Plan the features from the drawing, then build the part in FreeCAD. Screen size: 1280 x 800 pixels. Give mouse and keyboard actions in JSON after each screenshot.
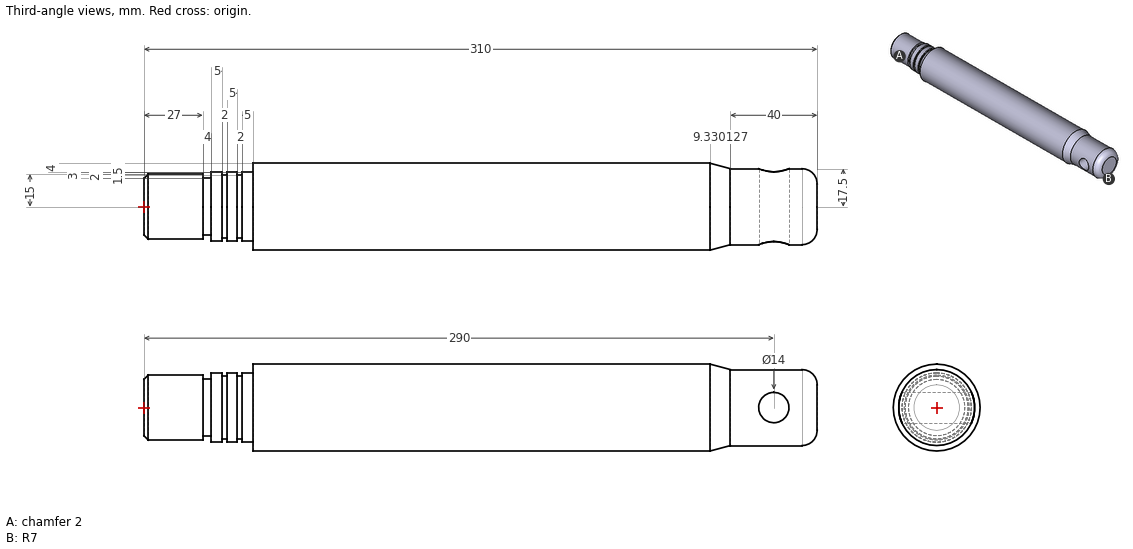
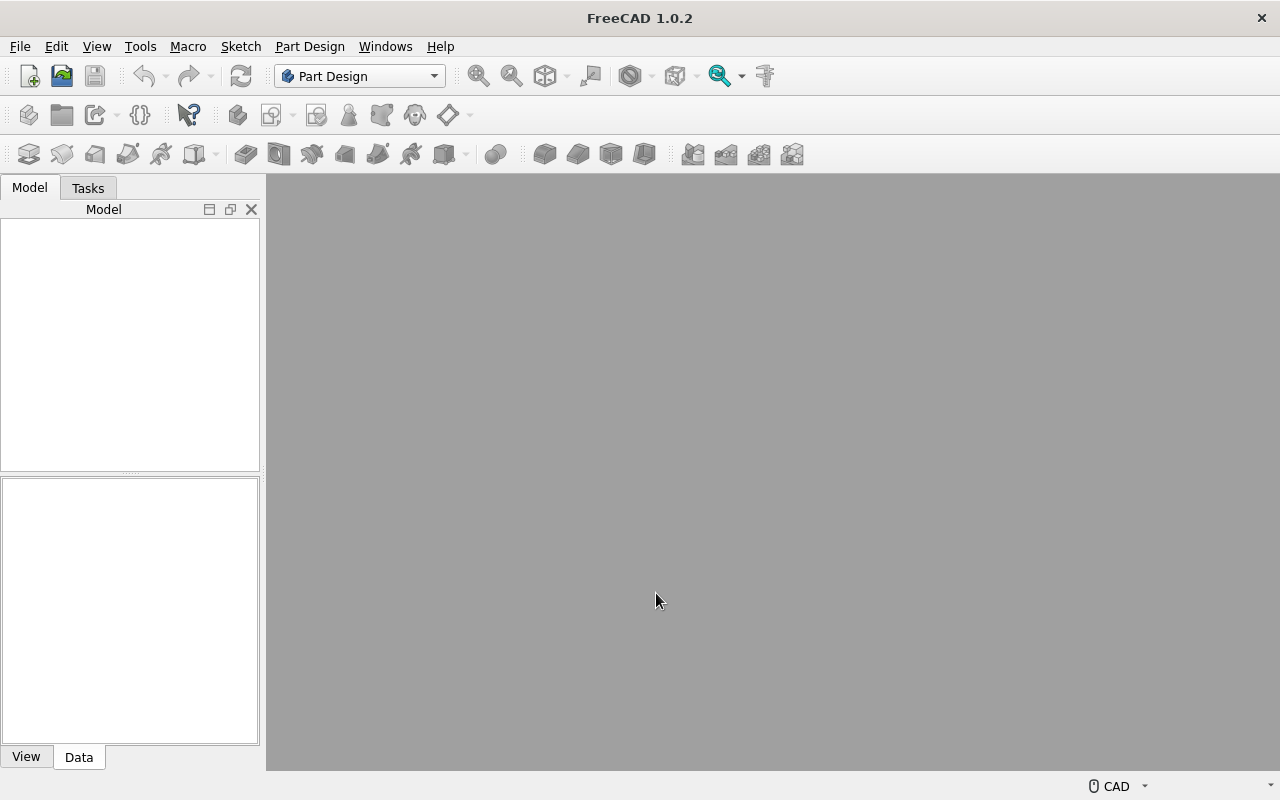
{"action": "key", "text": "ctrl+n"}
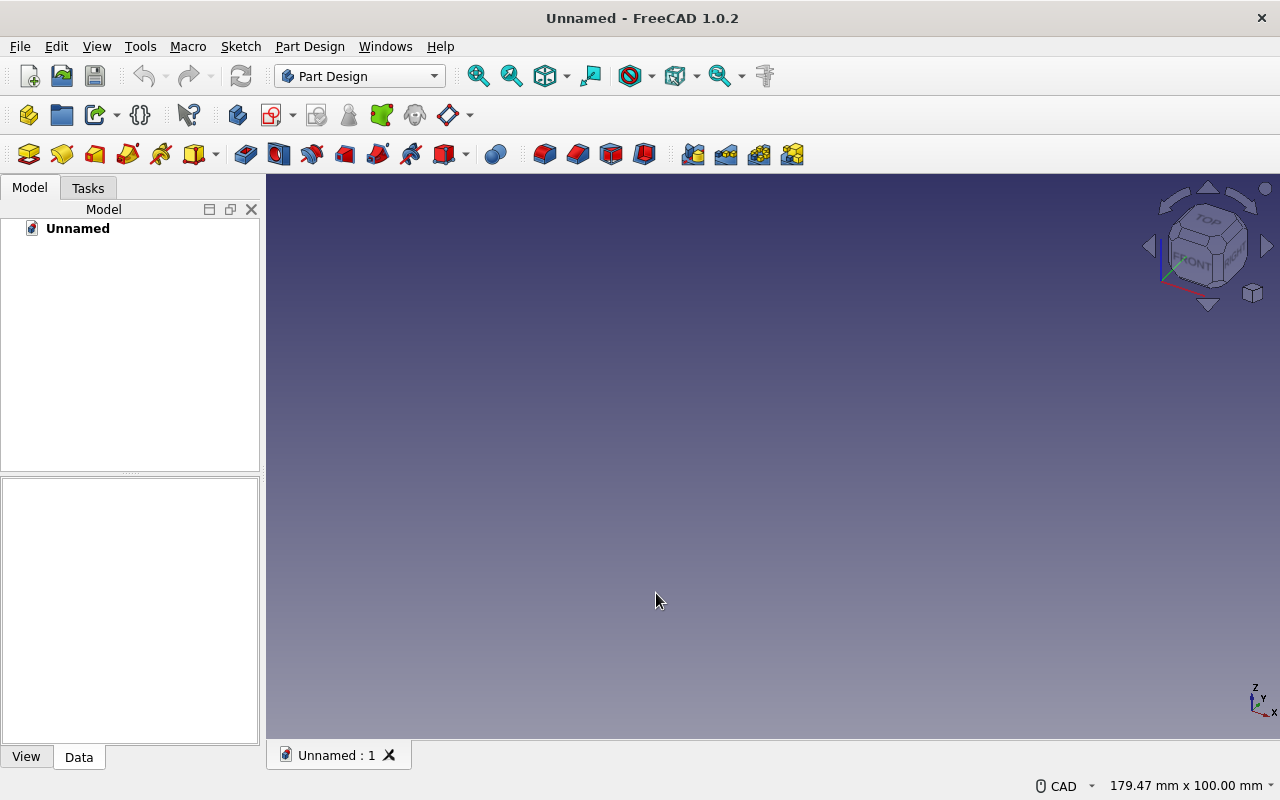
{"action": "left_click", "coordinate": [270, 116]}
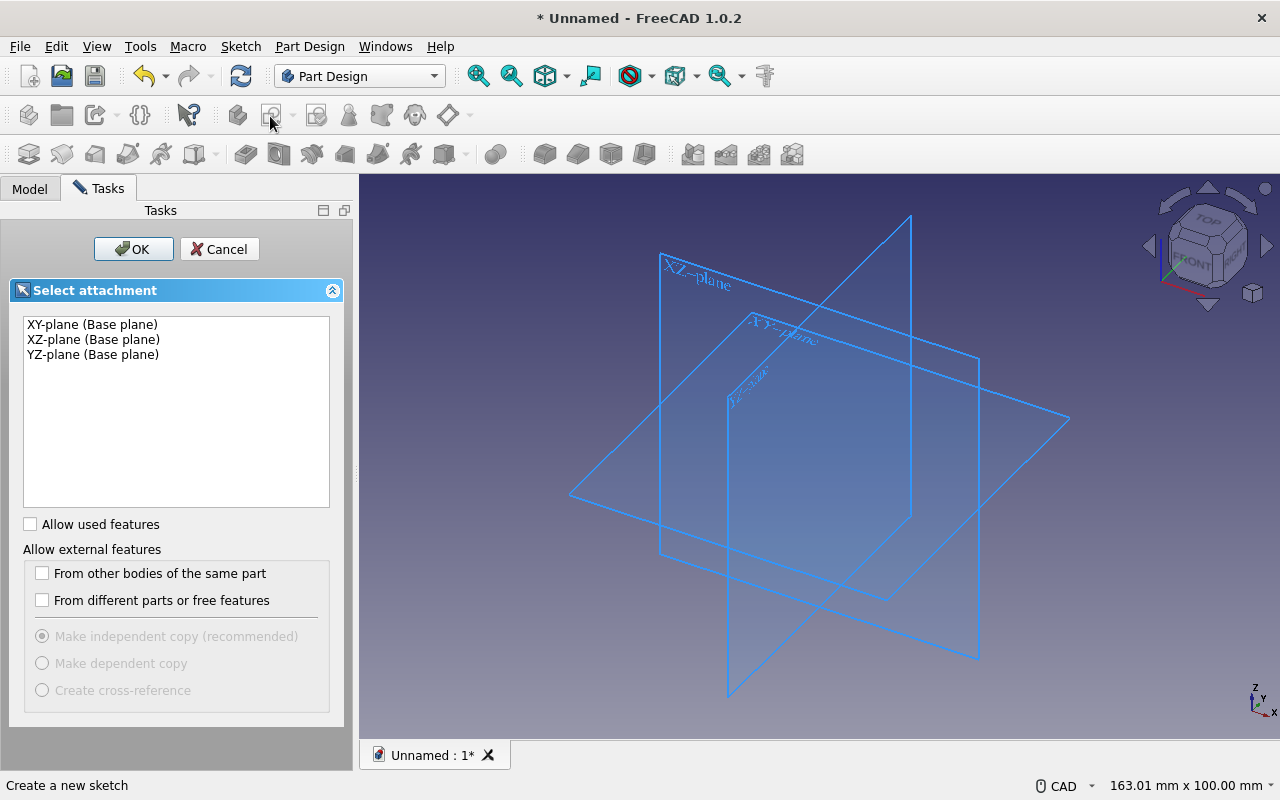
{"action": "left_click", "coordinate": [84, 324]}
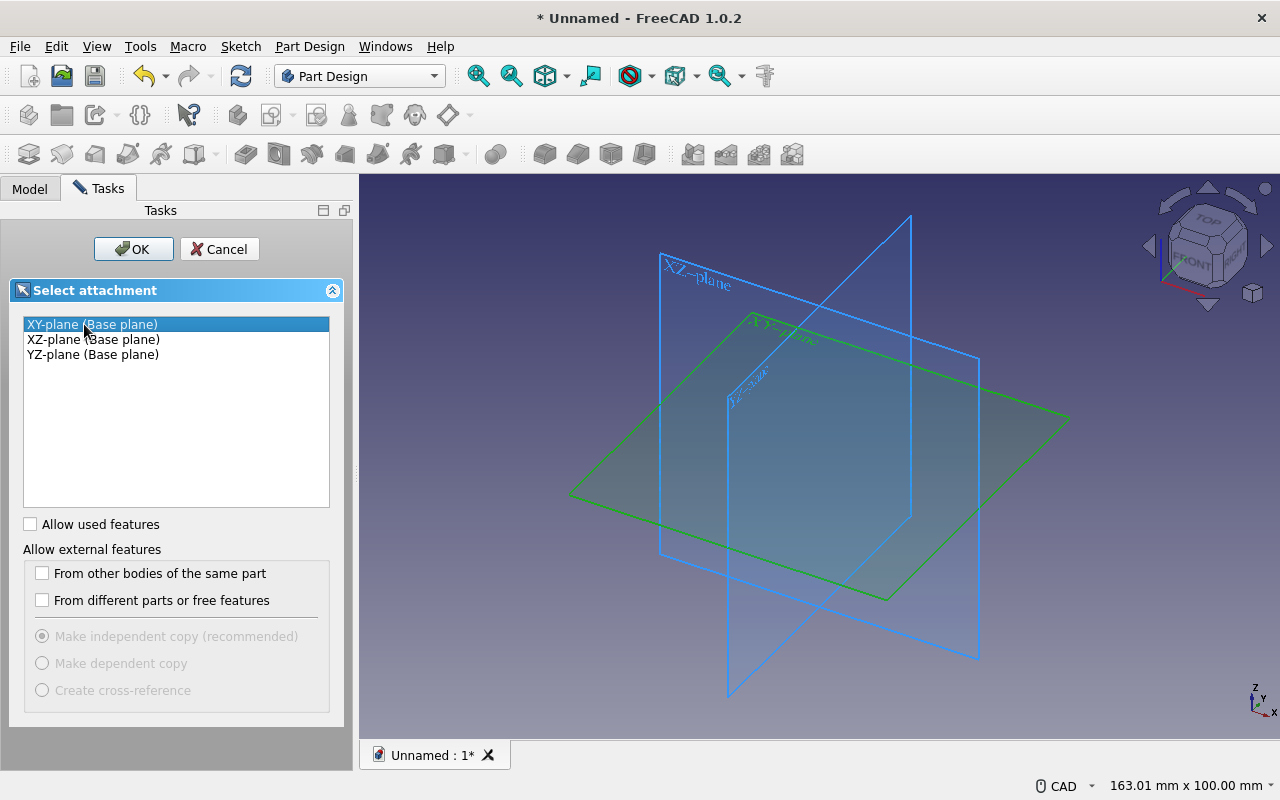
{"action": "left_click", "coordinate": [134, 249]}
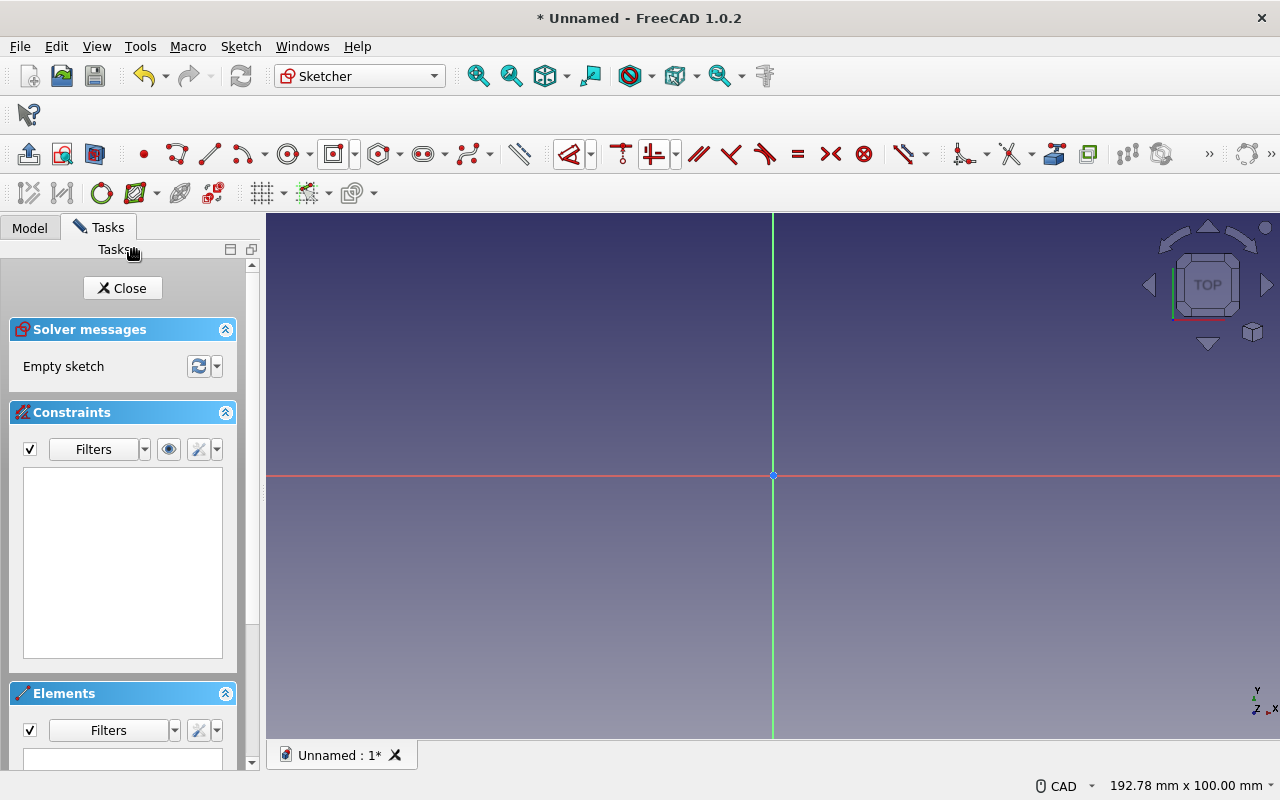
{"action": "scroll", "coordinate": [294, 507], "scroll_direction": "down", "scroll_amount": 5}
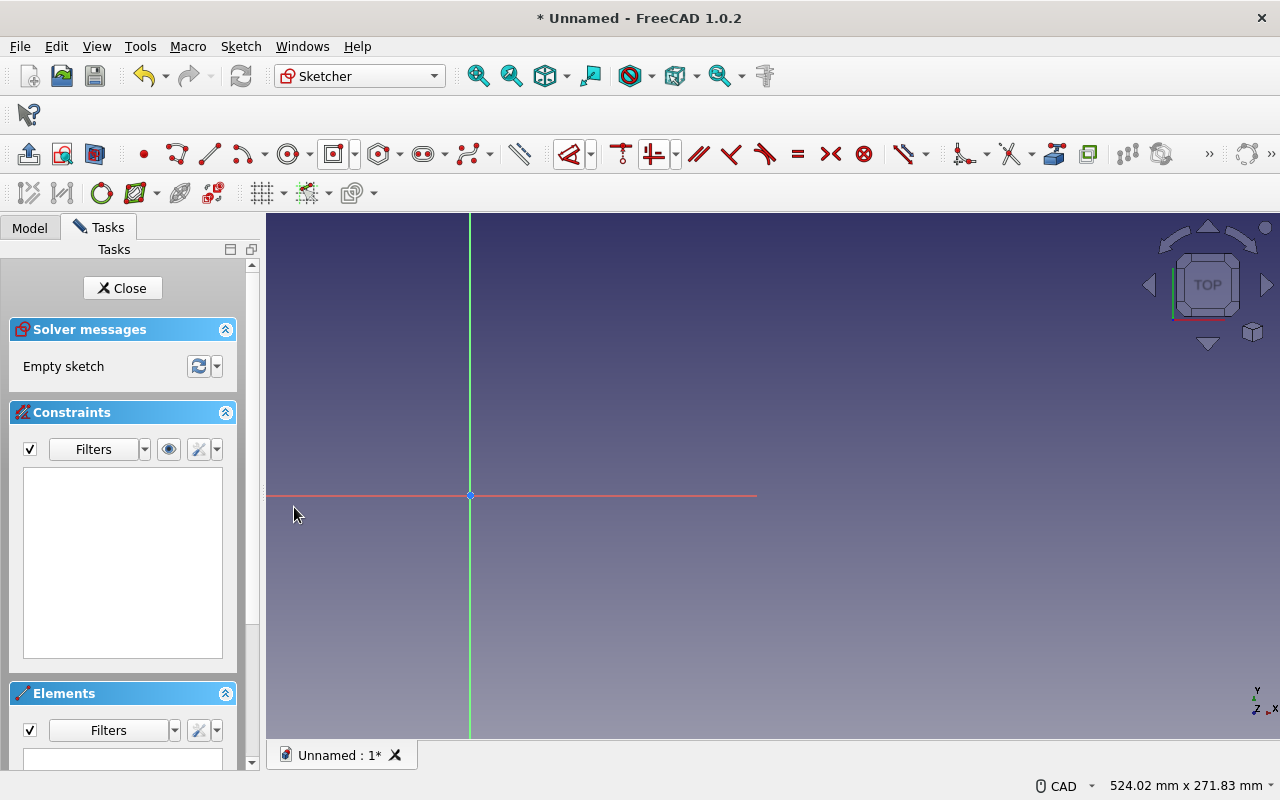
{"action": "left_click", "coordinate": [177, 154]}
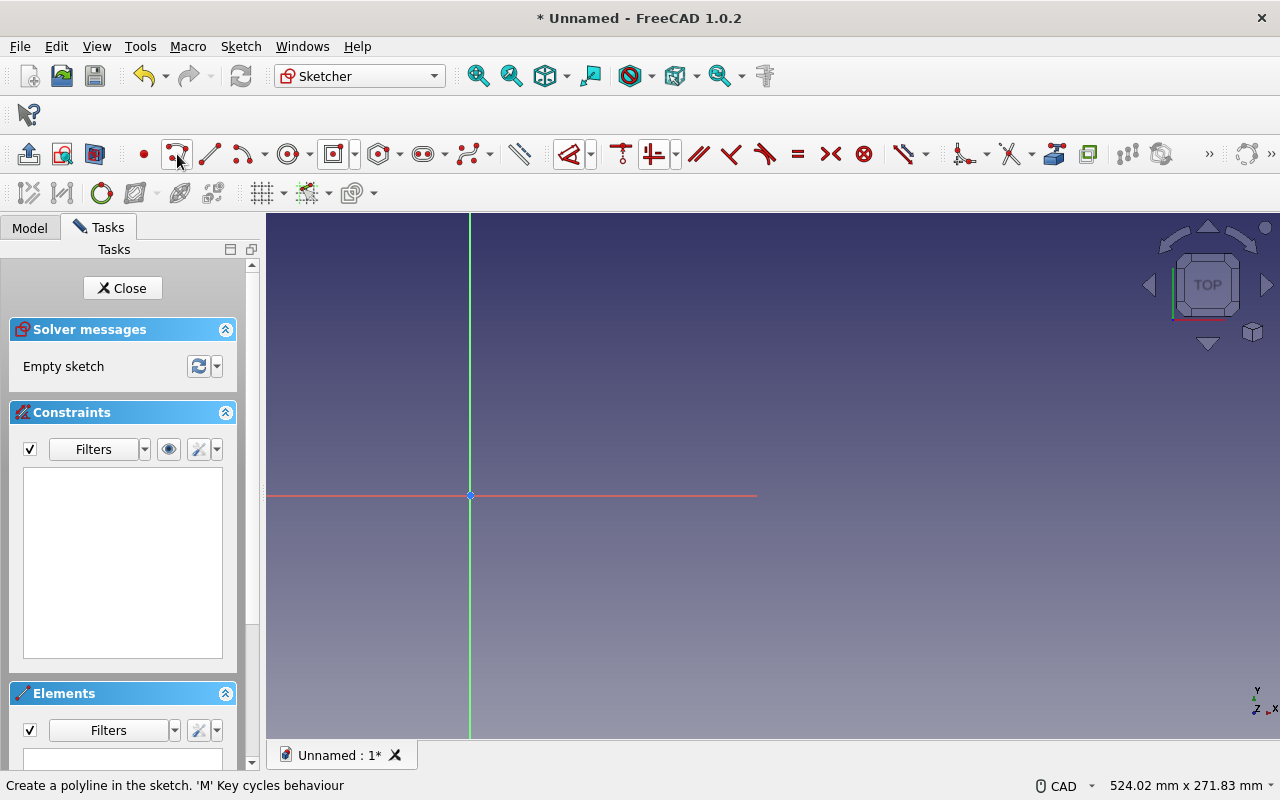
{"action": "left_click", "coordinate": [470, 496]}
{"action": "left_click", "coordinate": [1070, 487]}
{"action": "left_click", "coordinate": [1070, 462]}
{"action": "left_click", "coordinate": [993, 462]}
{"action": "left_click", "coordinate": [975, 457]}
{"action": "left_click", "coordinate": [567, 457]}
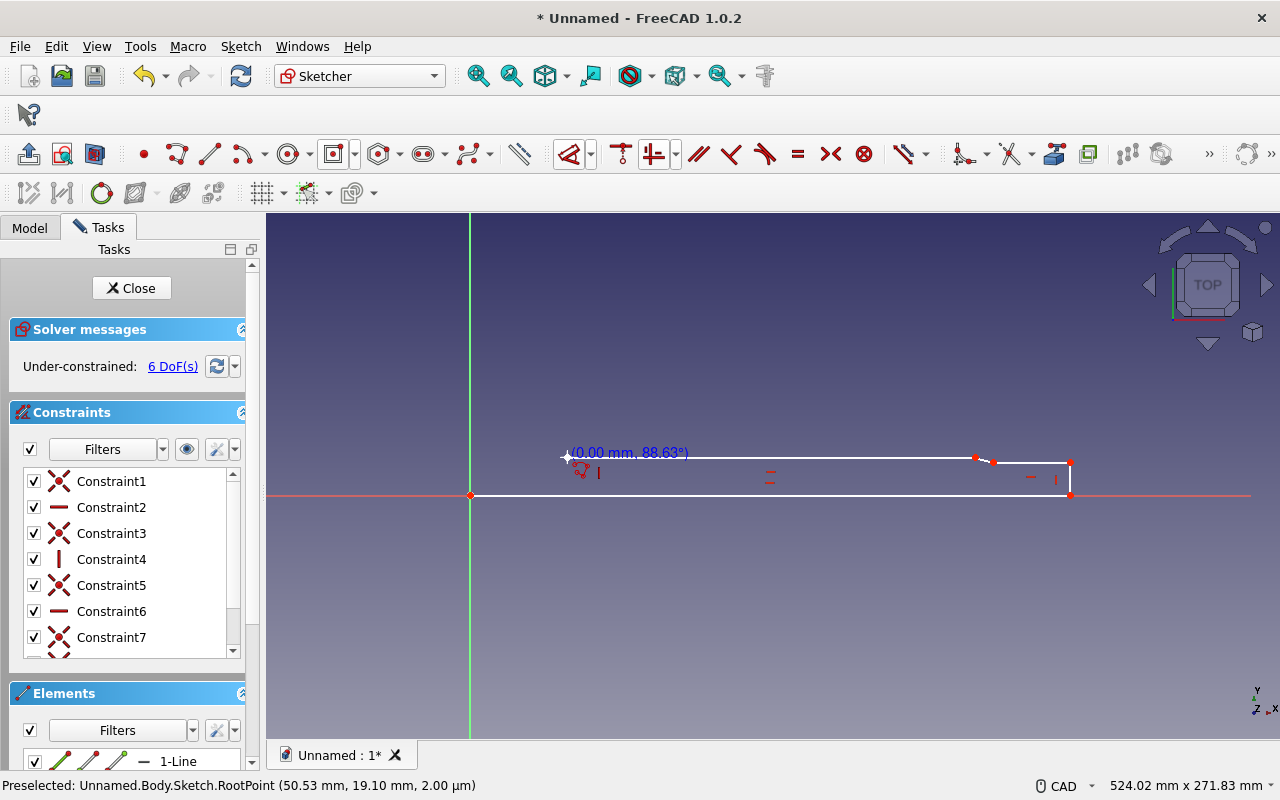
{"action": "scroll", "coordinate": [567, 465], "scroll_direction": "up", "scroll_amount": 4}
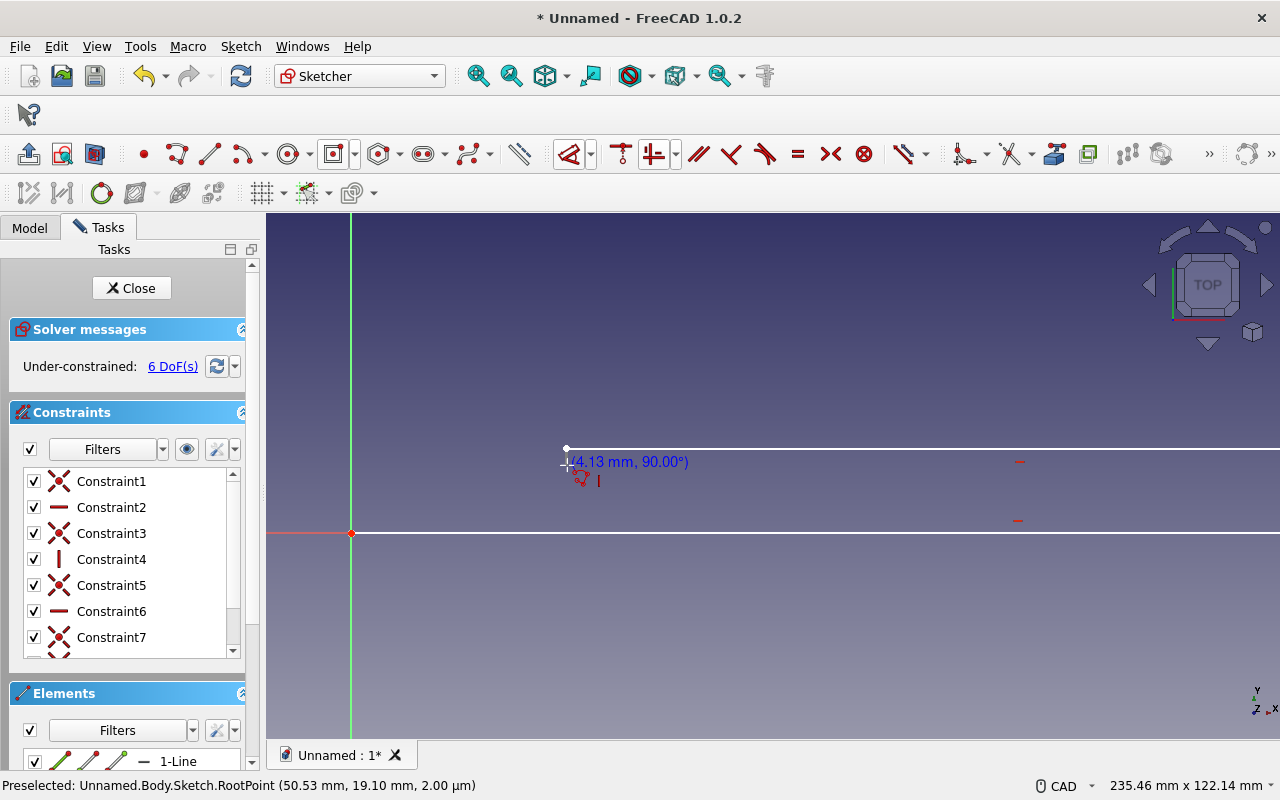
{"action": "left_click", "coordinate": [567, 464]}
{"action": "left_click", "coordinate": [545, 464]}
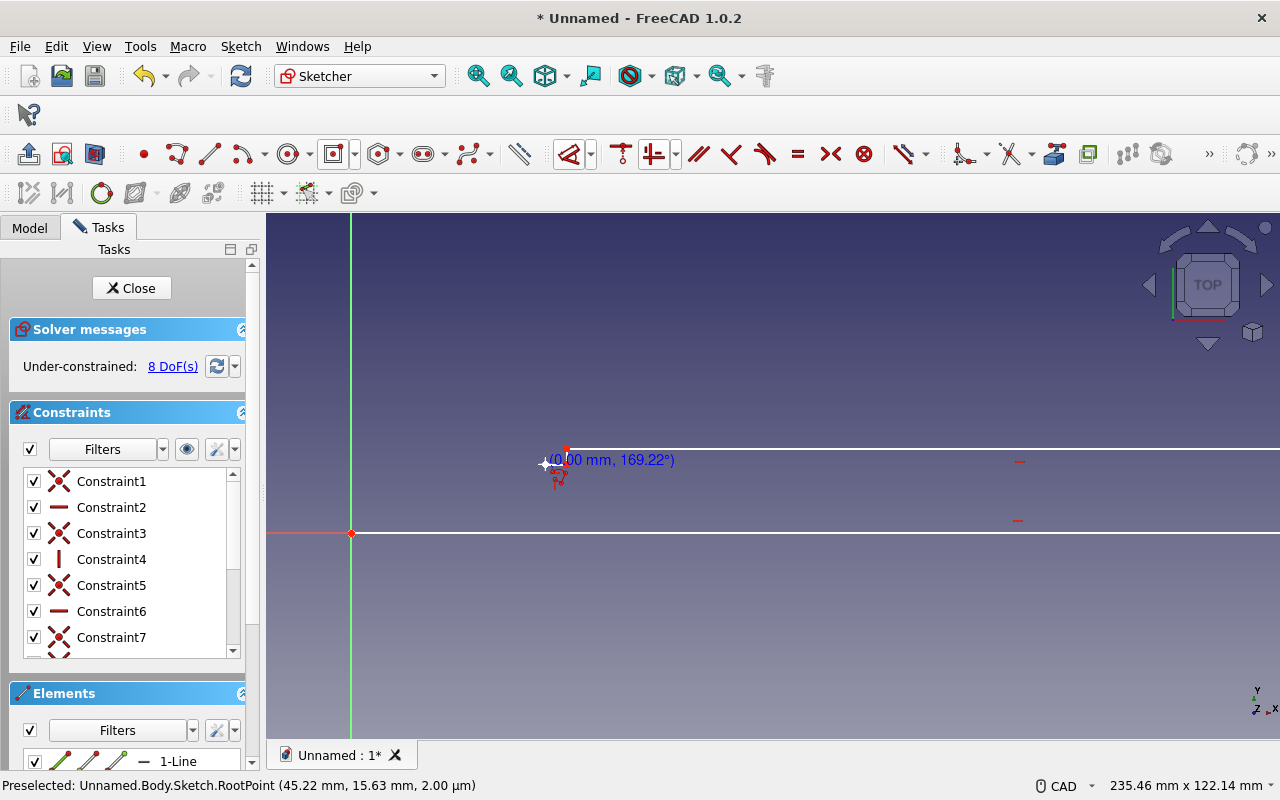
{"action": "scroll", "coordinate": [545, 471], "scroll_direction": "up", "scroll_amount": 5}